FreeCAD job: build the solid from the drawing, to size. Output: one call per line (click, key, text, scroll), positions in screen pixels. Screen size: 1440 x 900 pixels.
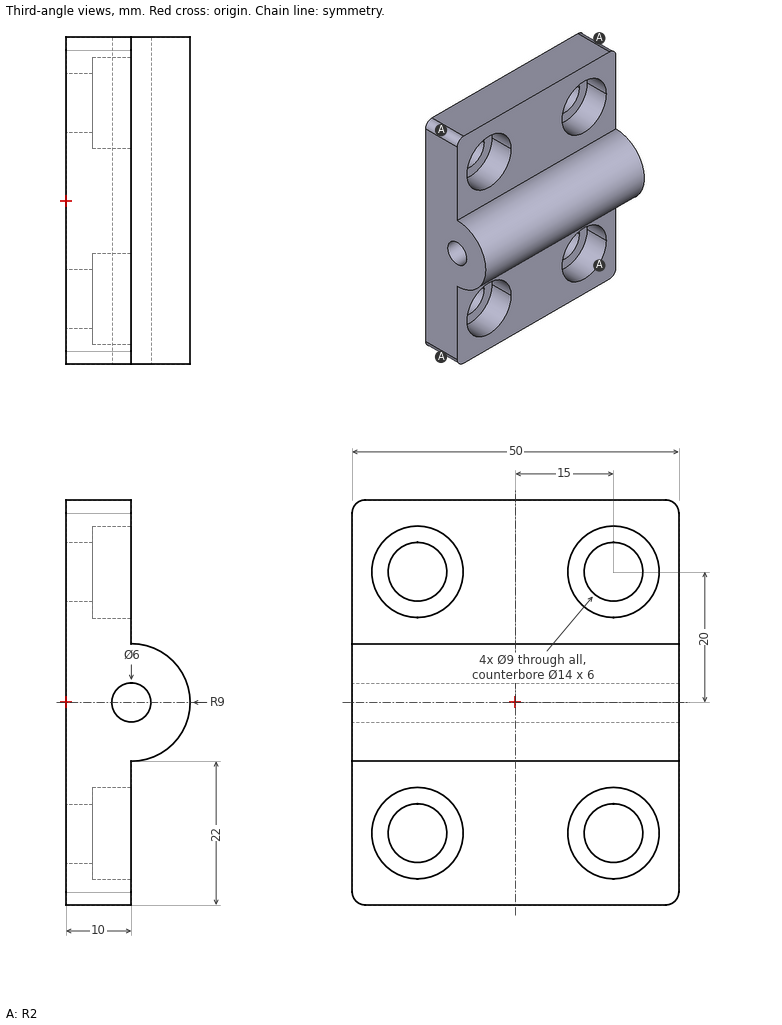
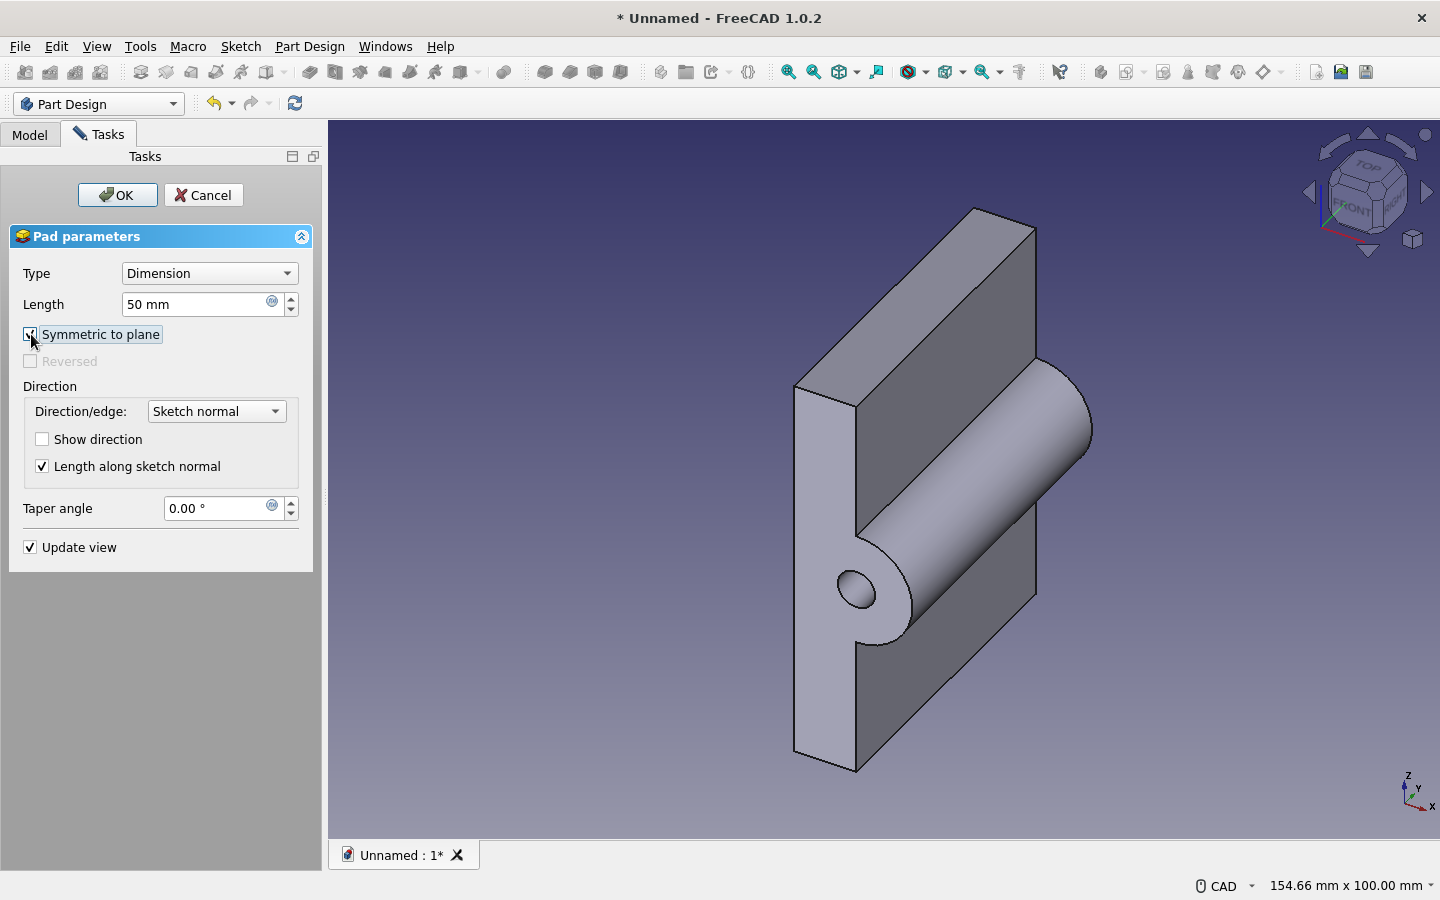
click(118, 195)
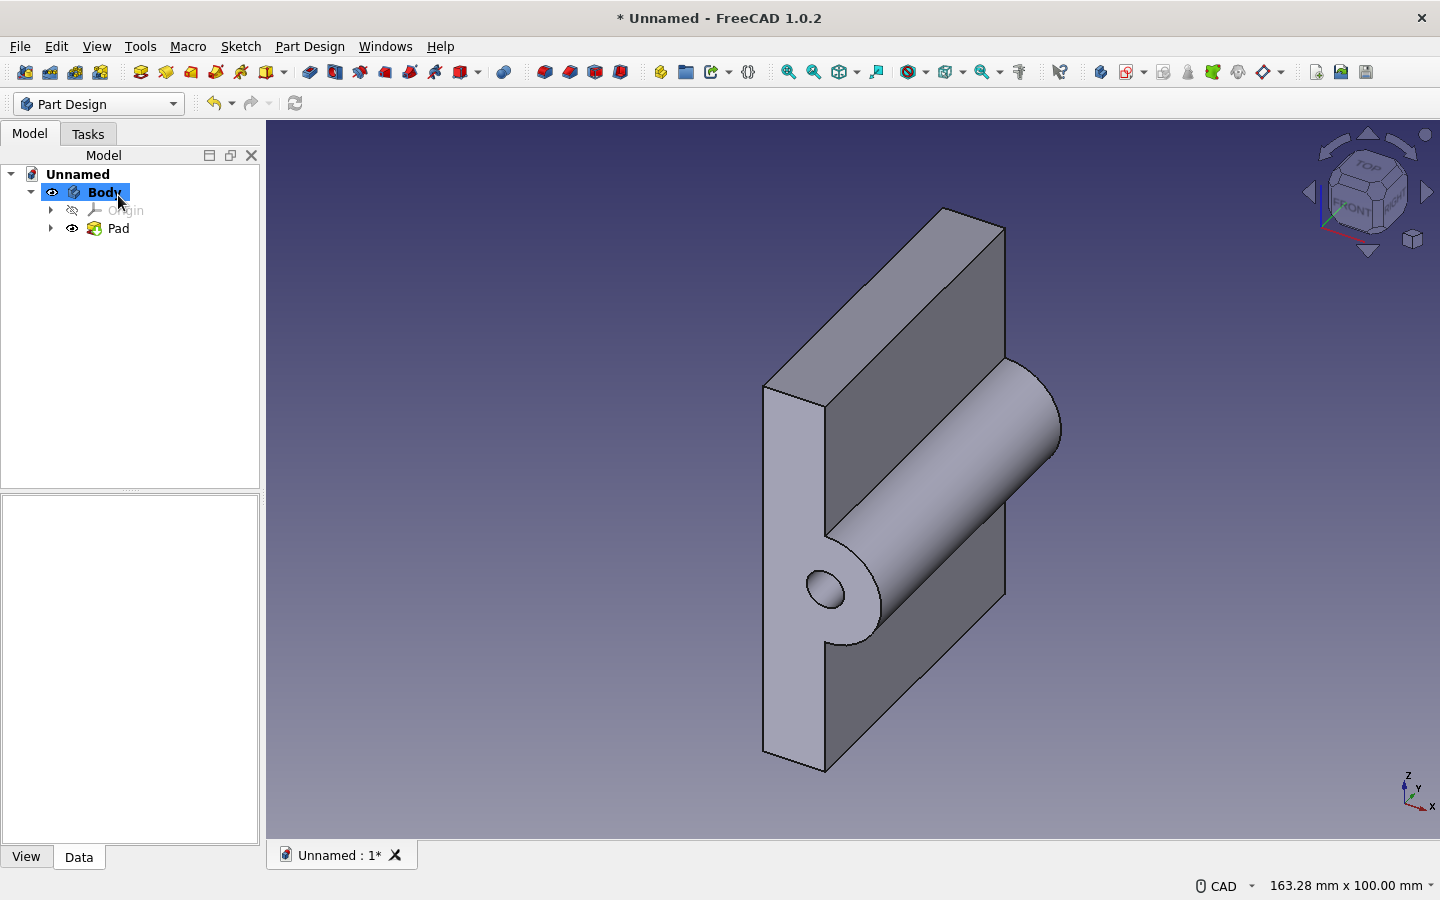
click(890, 407)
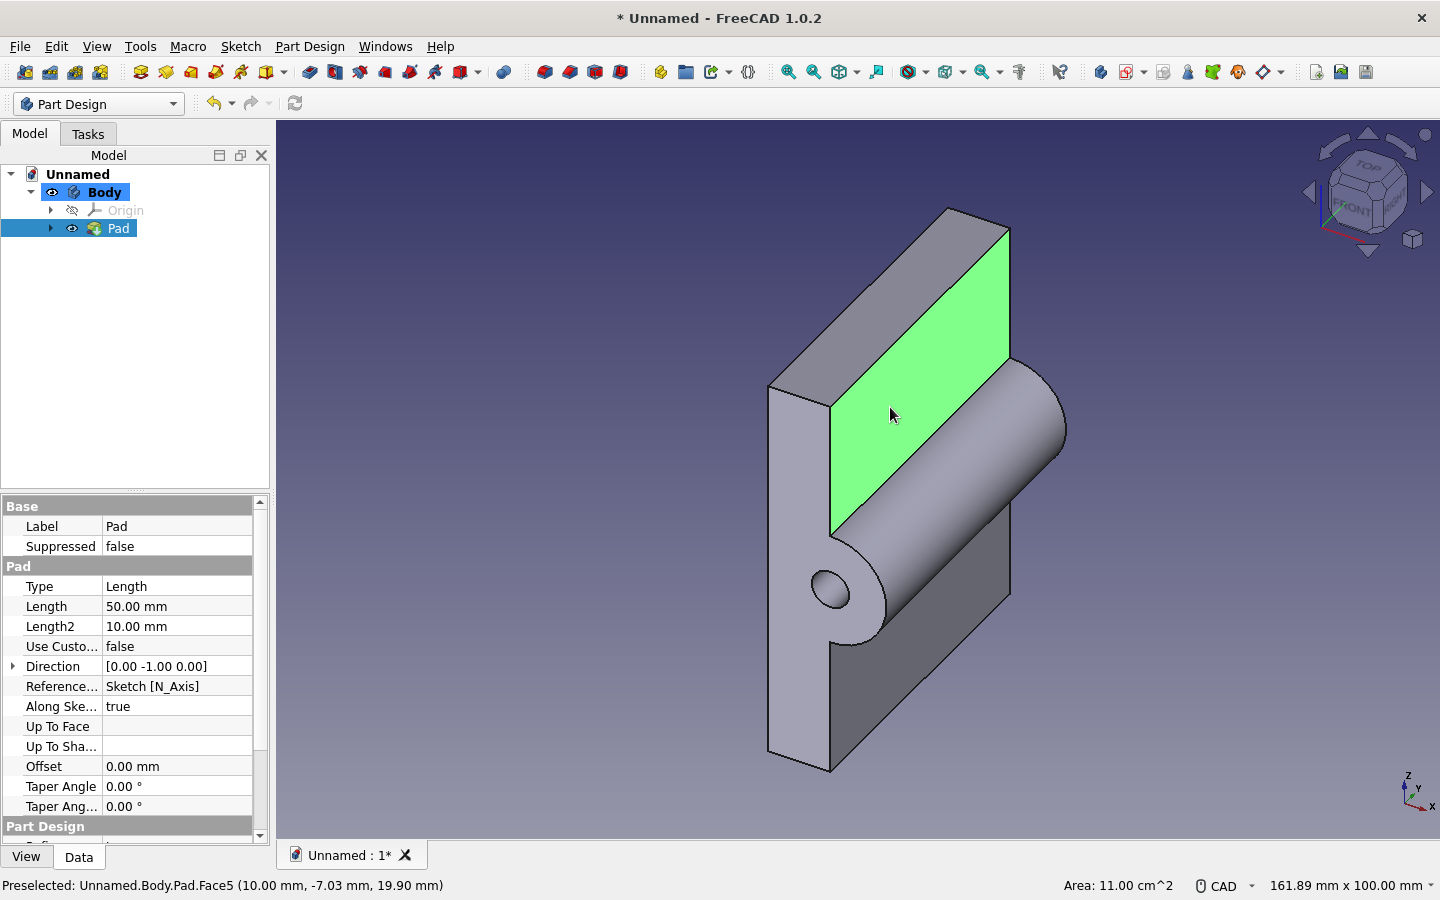
click(1126, 72)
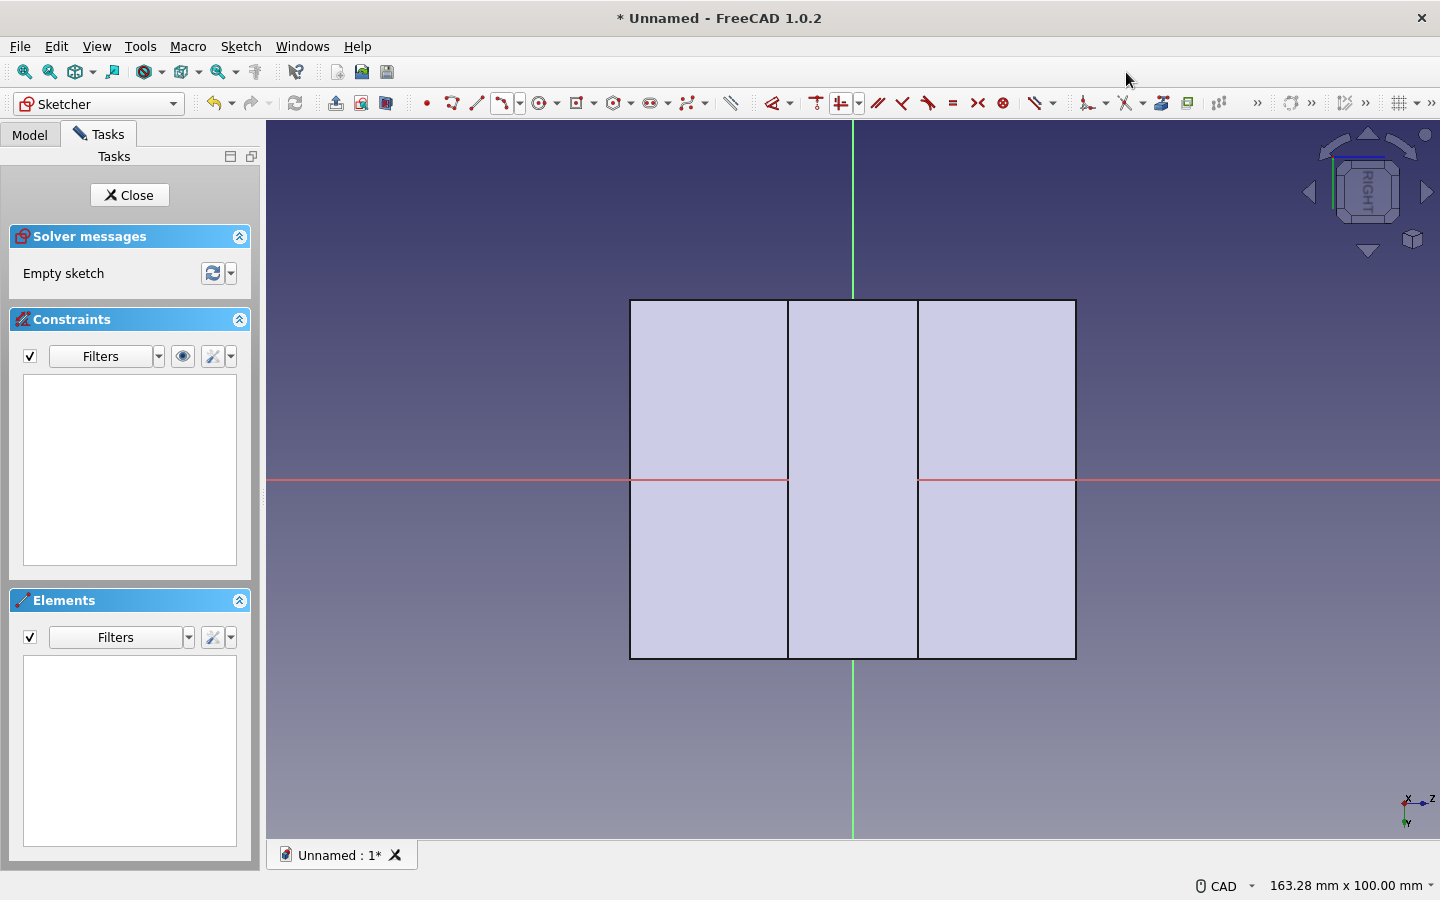
click(386, 104)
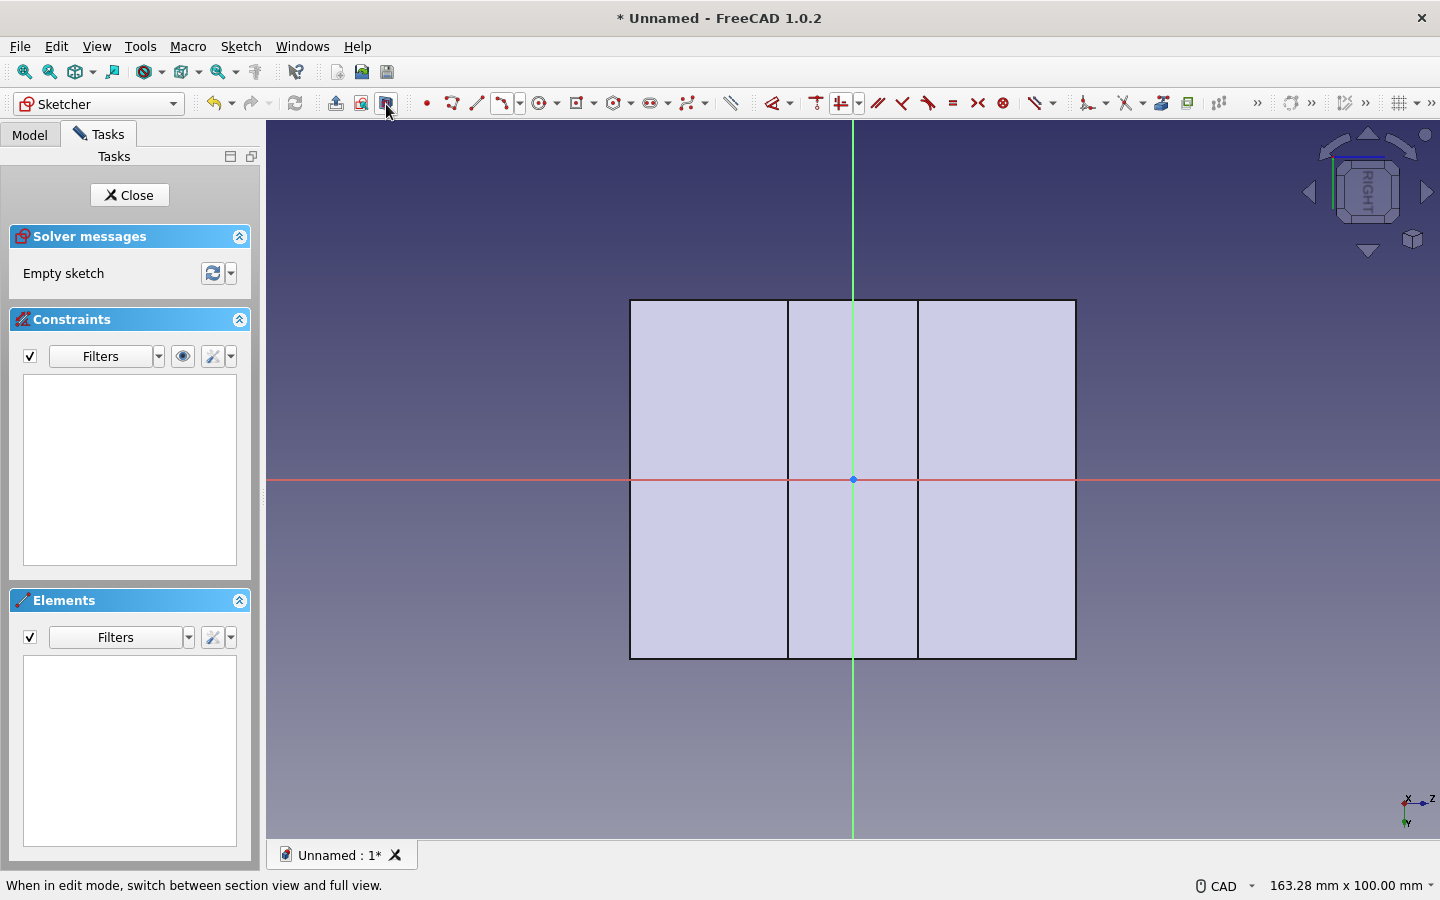
scroll(936, 480, up, 3)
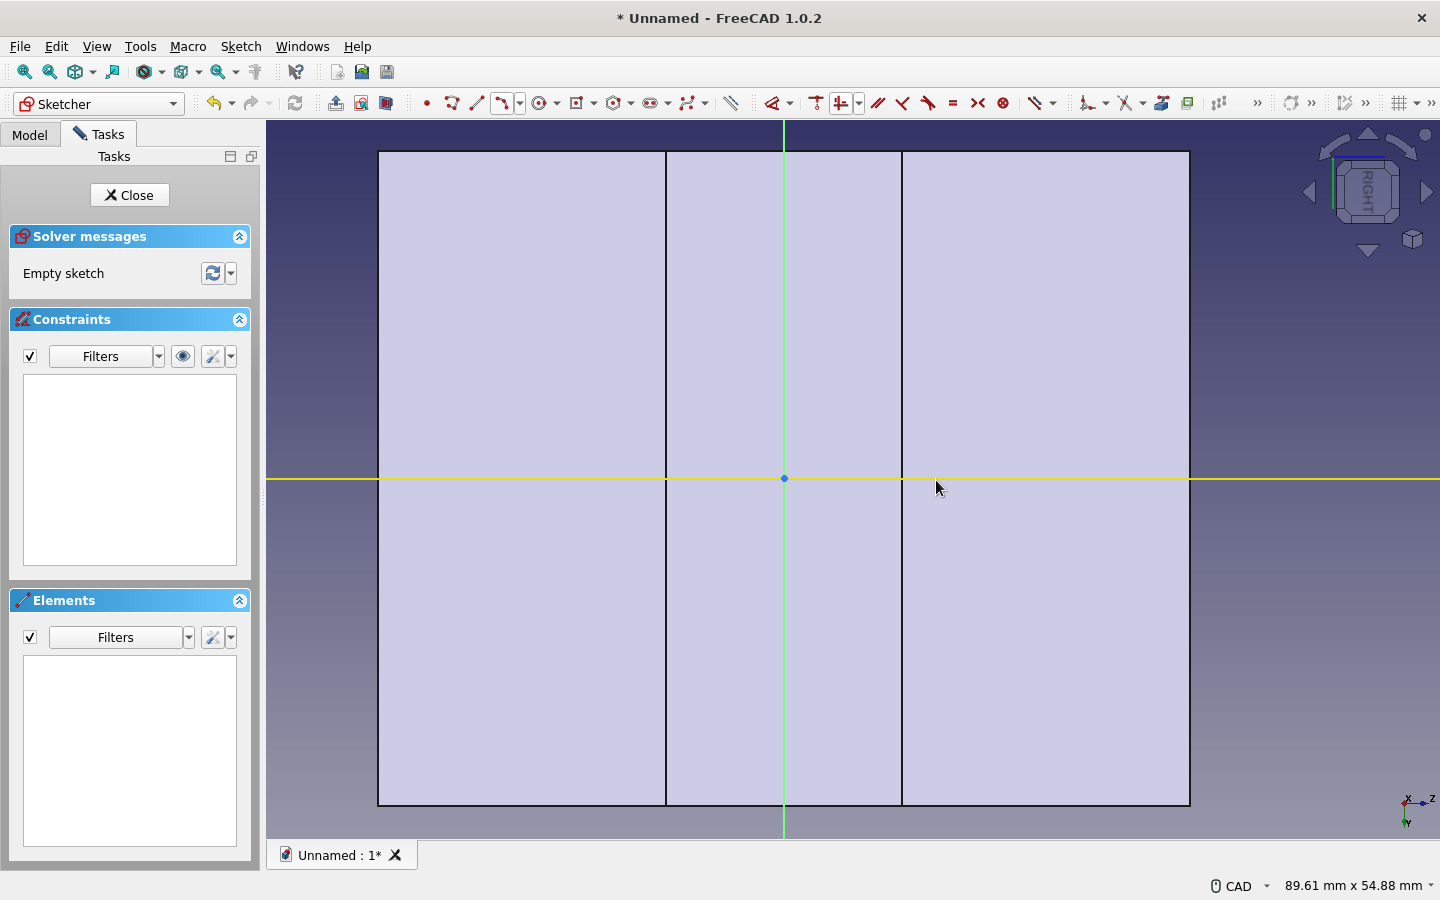
click(538, 104)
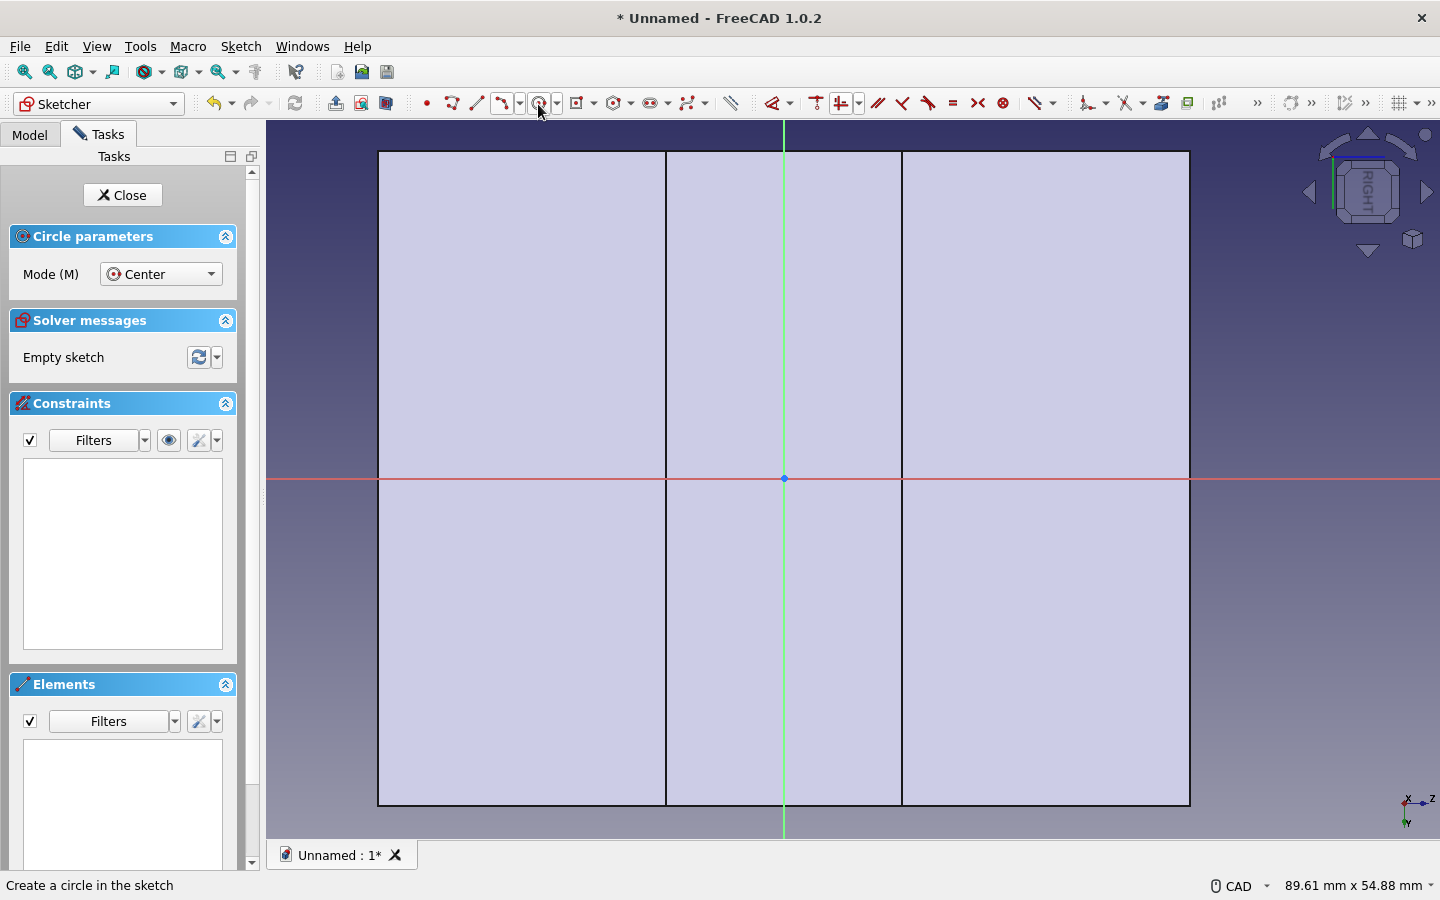
click(1046, 675)
move(1088, 634)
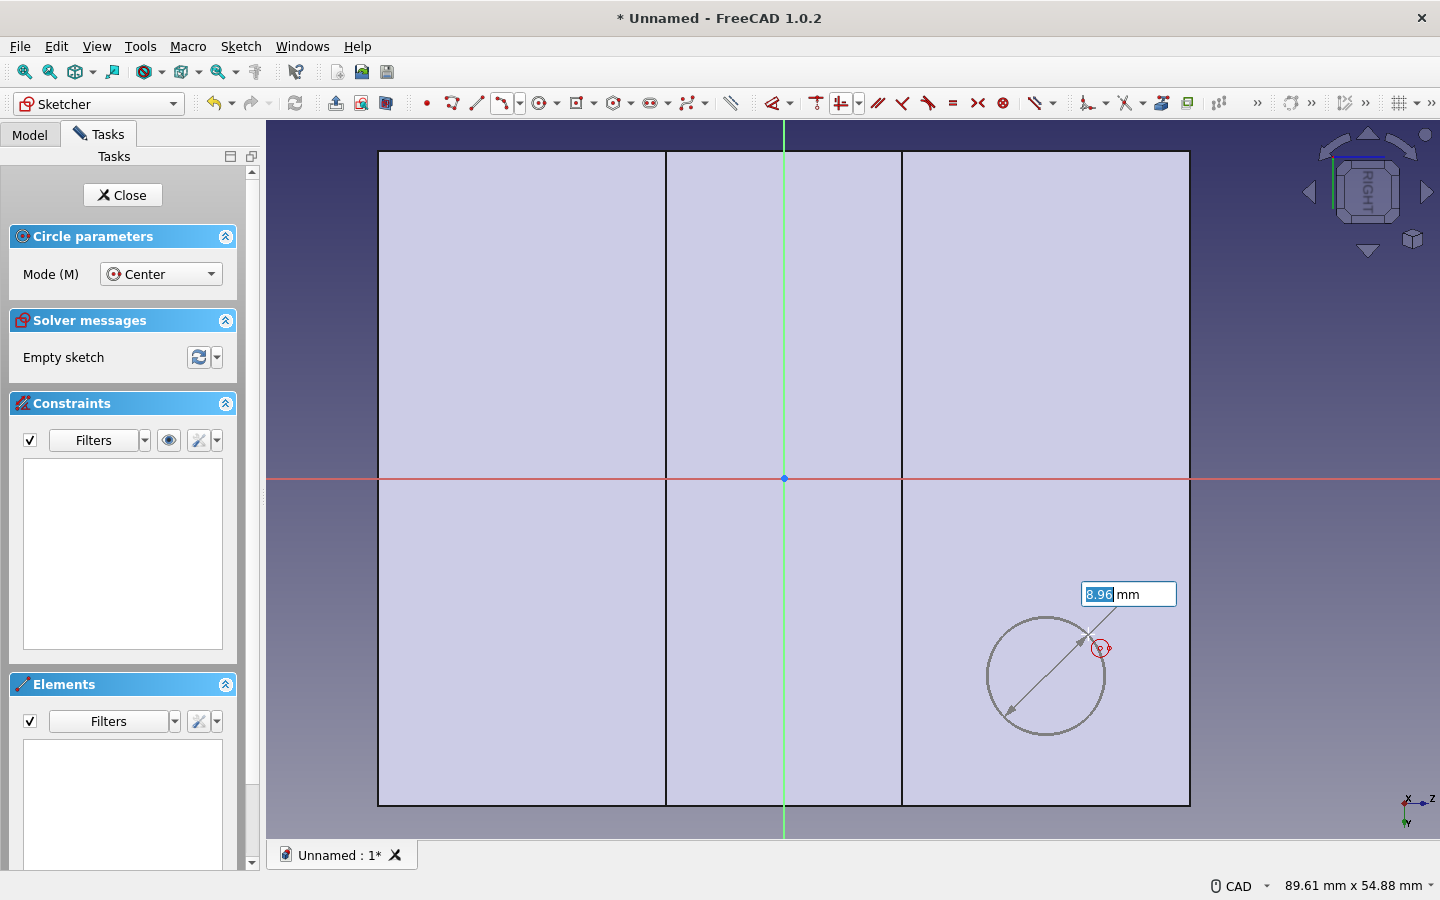
text(9)
key(Return)